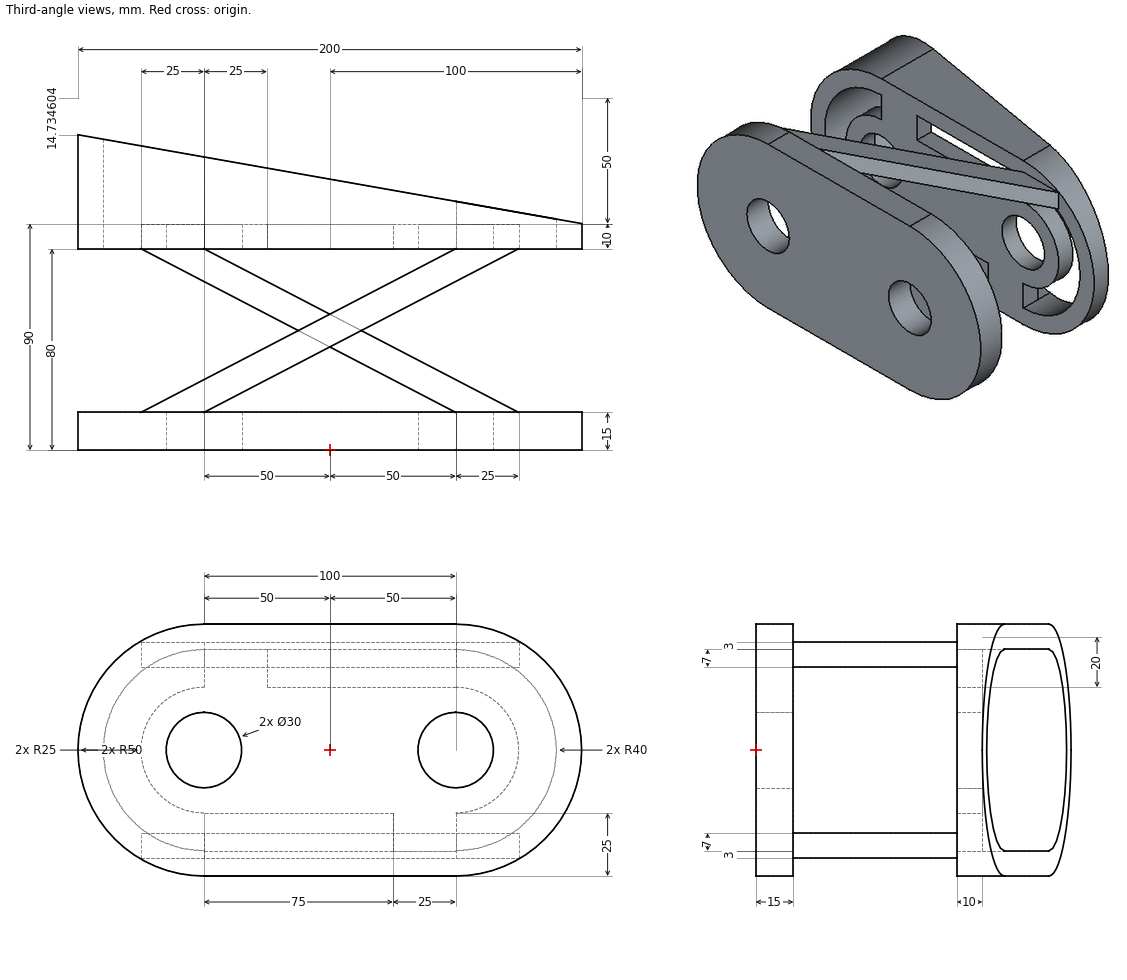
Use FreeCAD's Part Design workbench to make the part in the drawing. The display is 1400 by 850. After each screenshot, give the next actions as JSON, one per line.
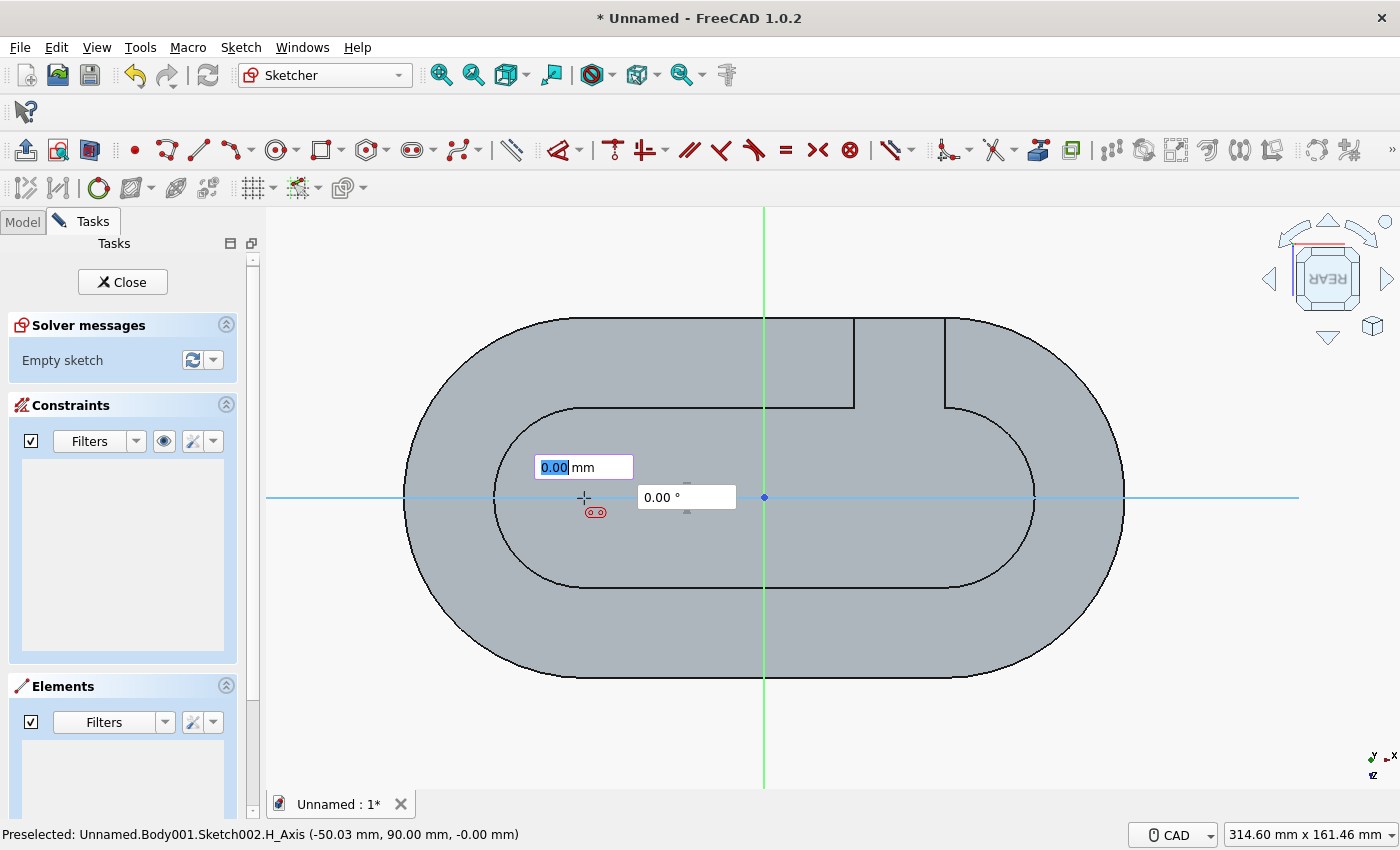
{"action": "left_click", "coordinate": [945, 489]}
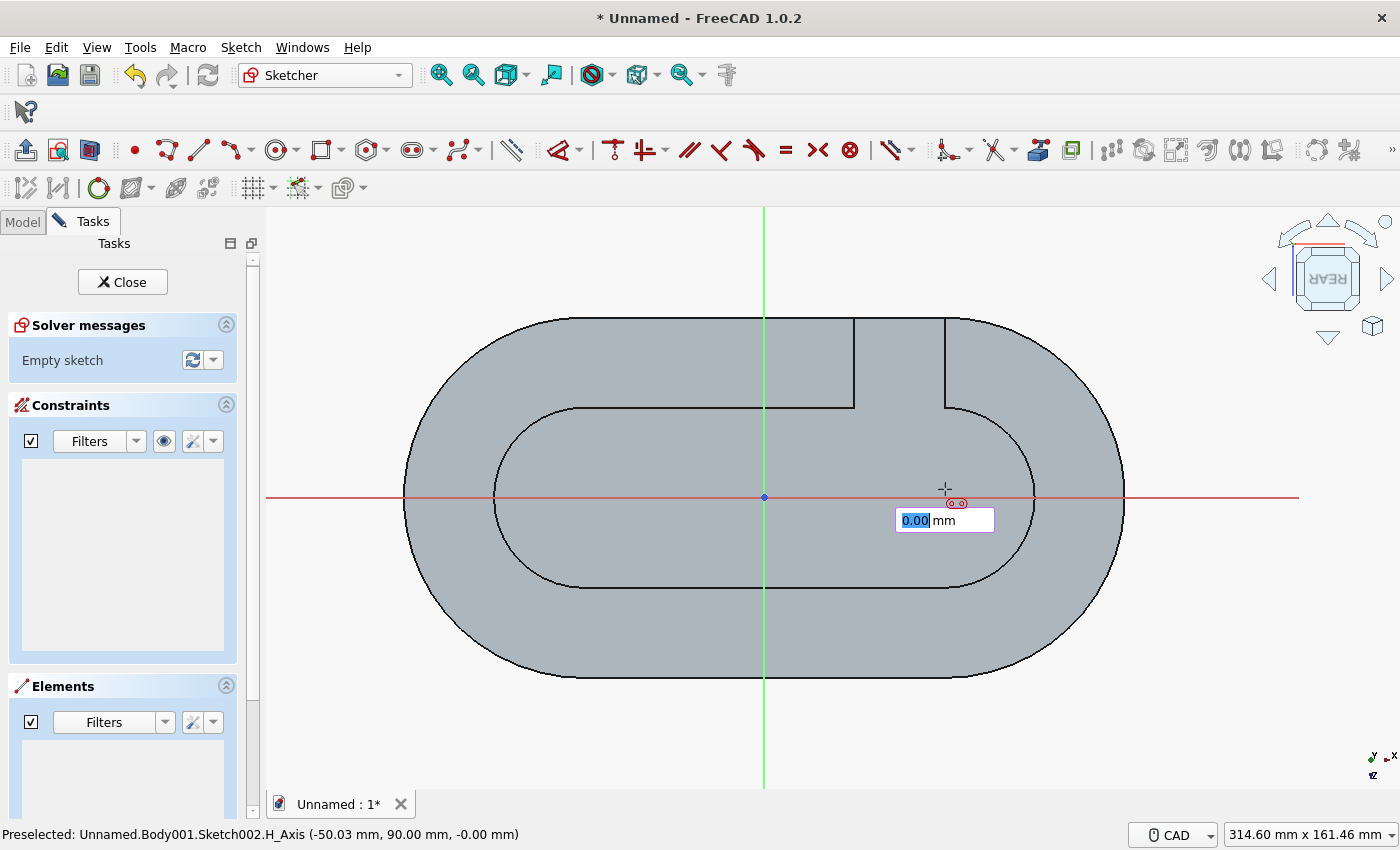
{"action": "left_click", "coordinate": [818, 318]}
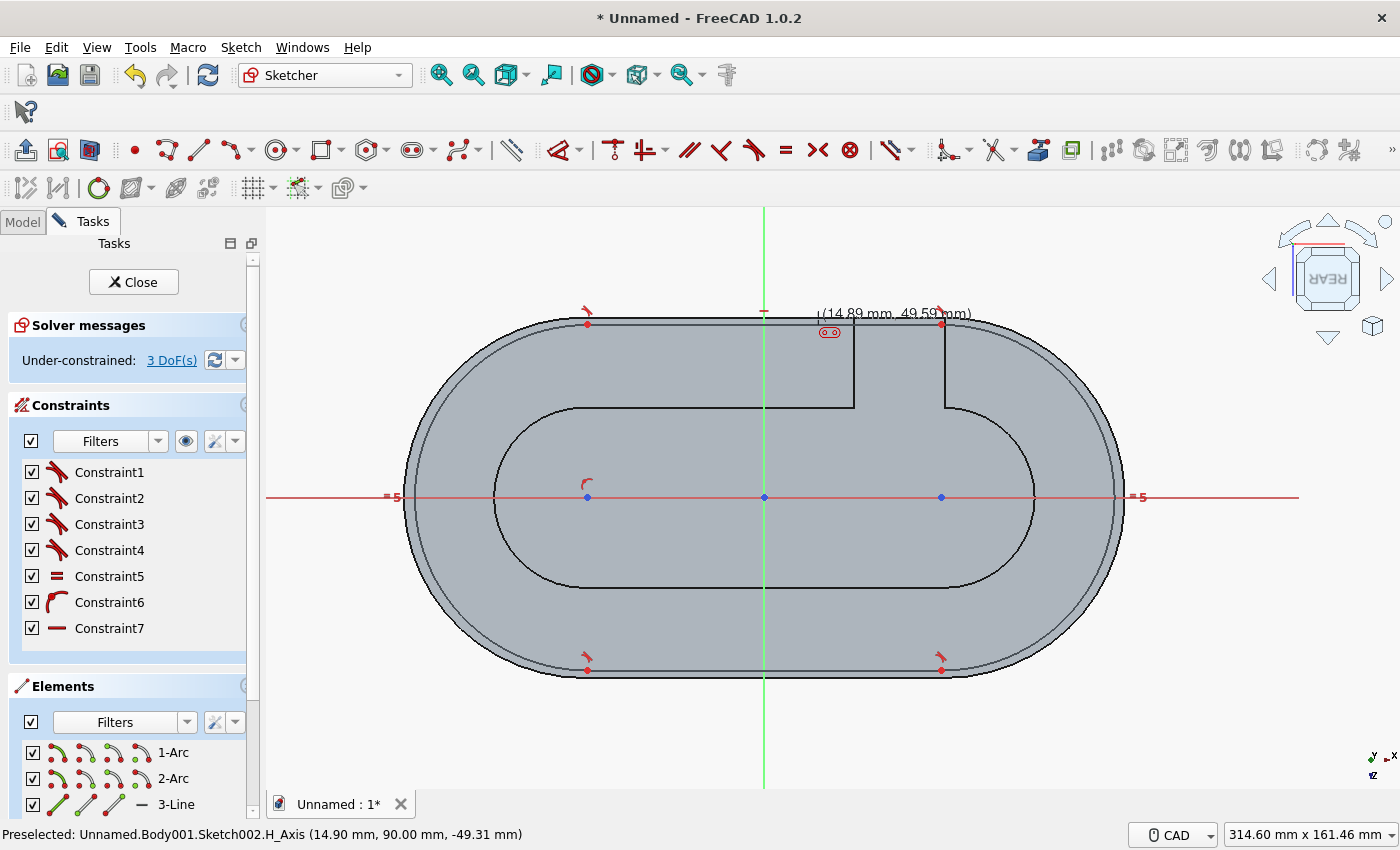
{"action": "left_click", "coordinate": [588, 498]}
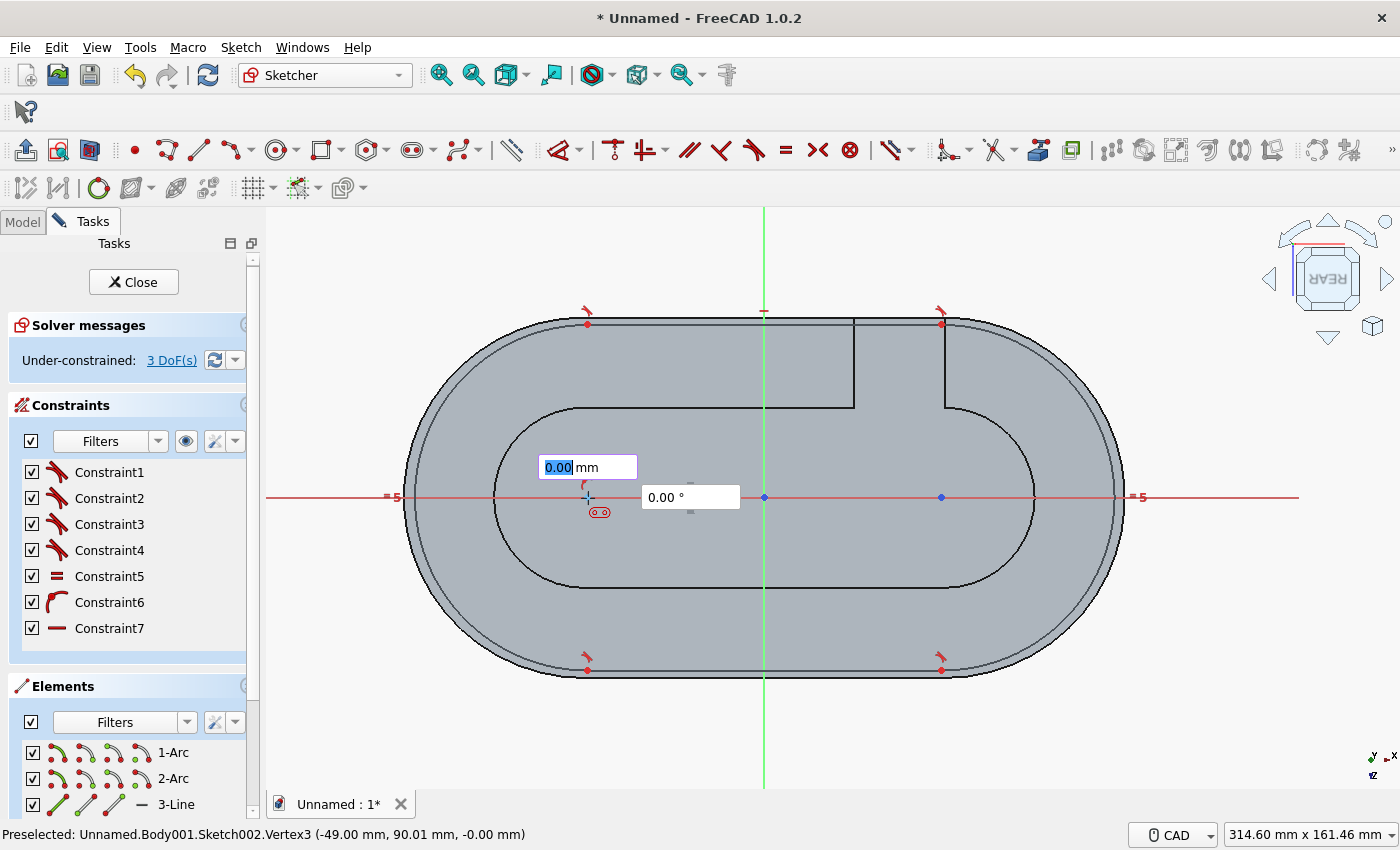
{"action": "left_click", "coordinate": [945, 489]}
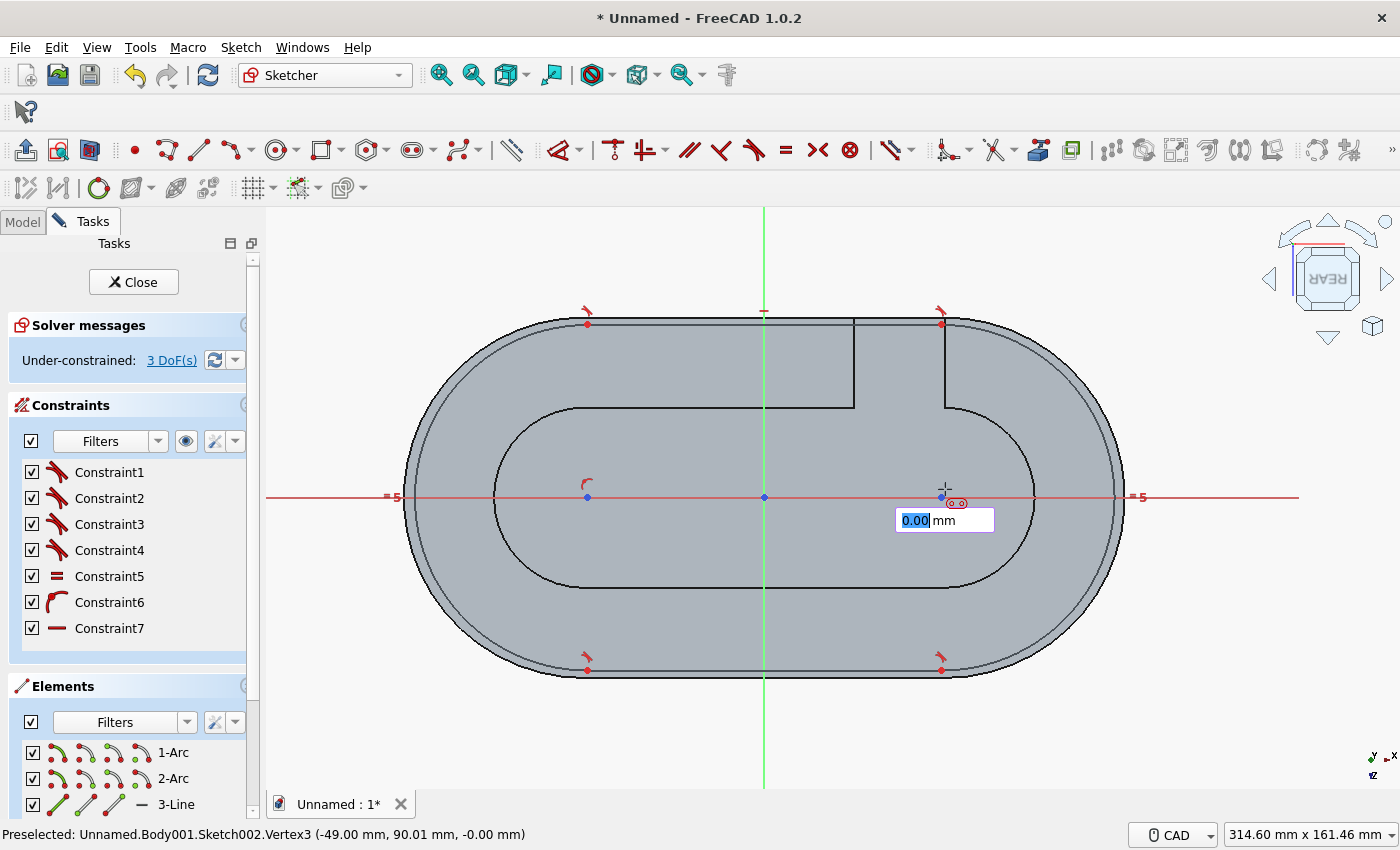
{"action": "left_click", "coordinate": [710, 354]}
{"action": "key", "text": "Escape"}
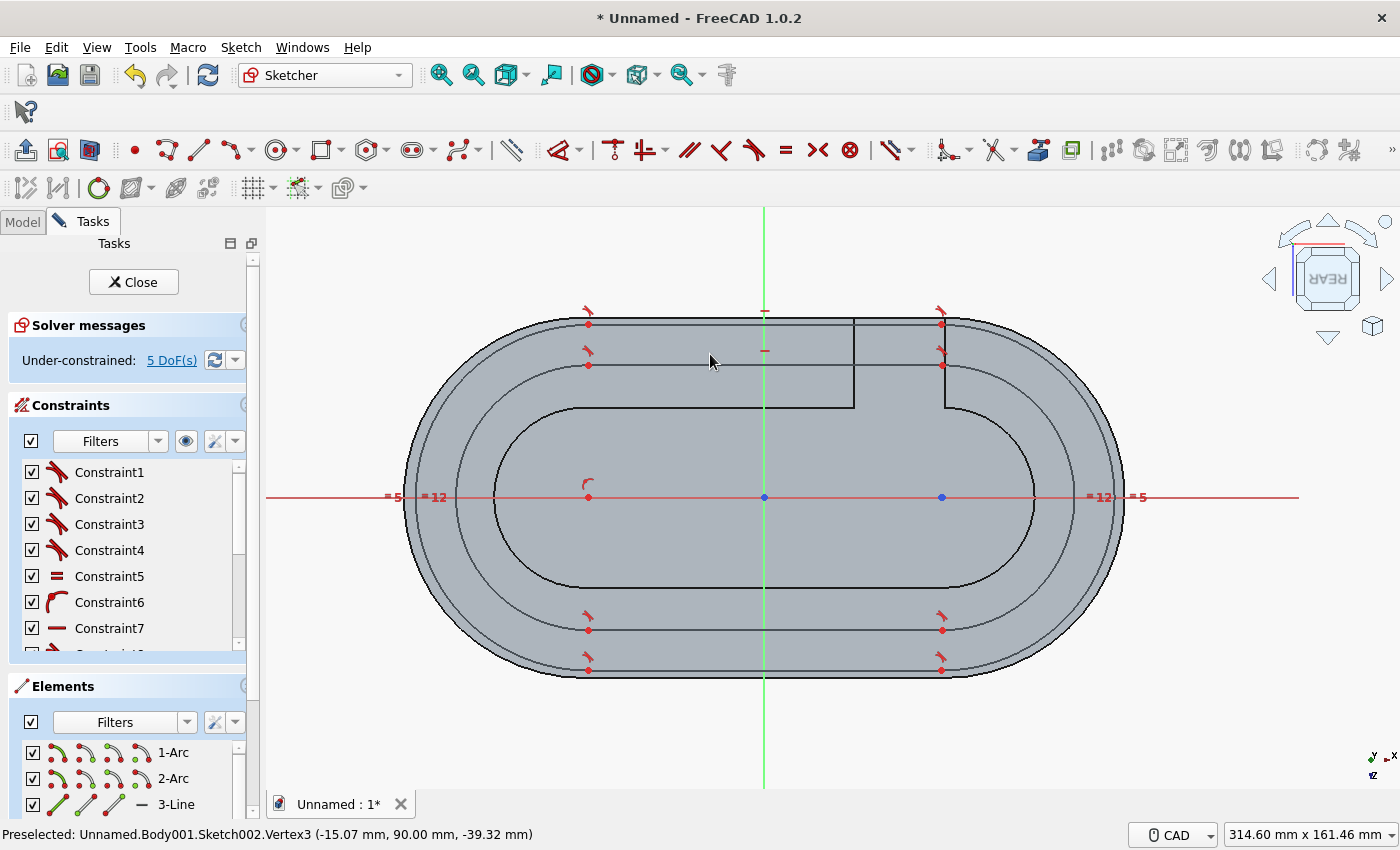
{"action": "left_click", "coordinate": [558, 150]}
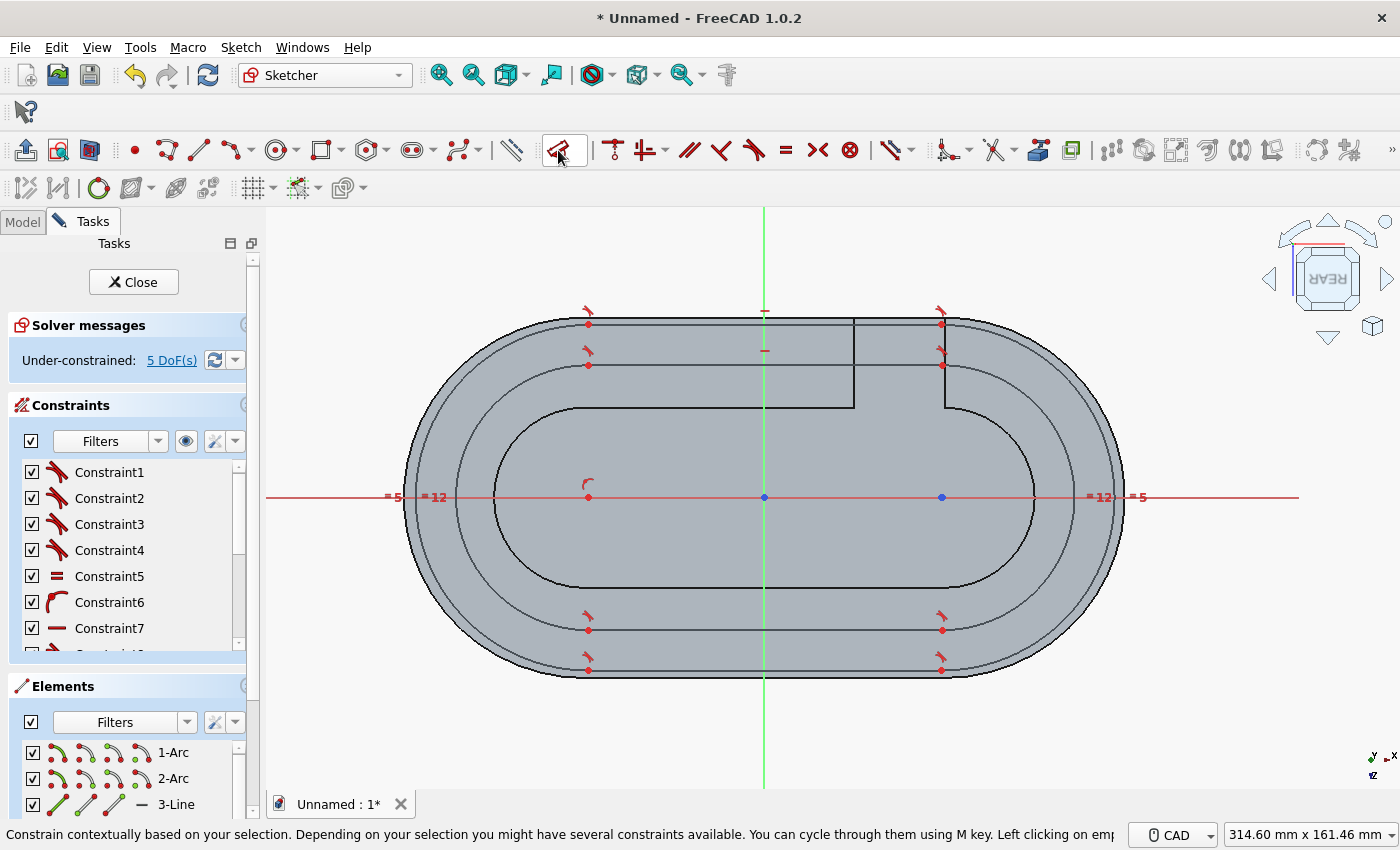
{"action": "left_click", "coordinate": [449, 396]}
{"action": "left_click", "coordinate": [423, 377]}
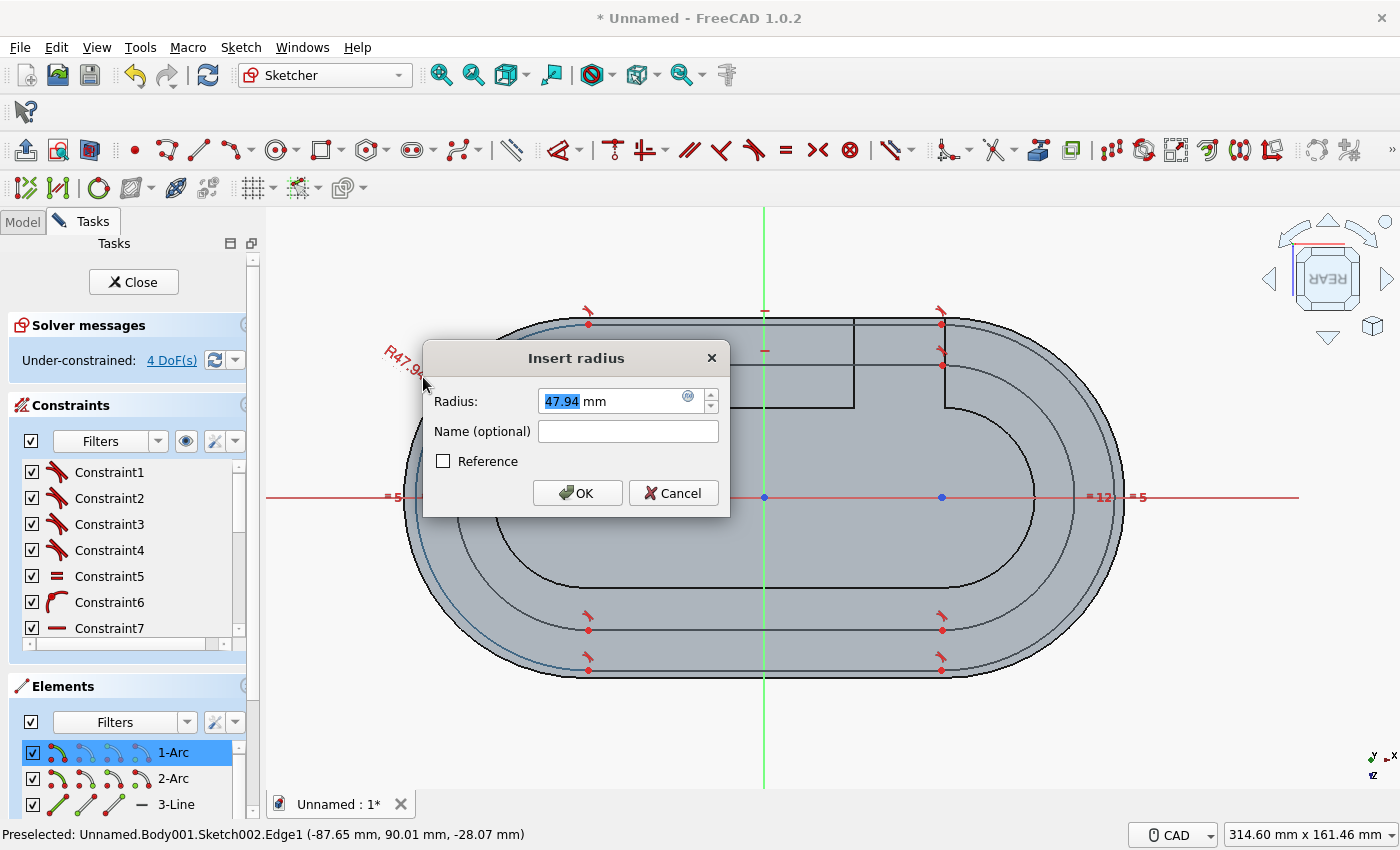
{"action": "type", "text": "50"}
{"action": "key", "text": "Return"}